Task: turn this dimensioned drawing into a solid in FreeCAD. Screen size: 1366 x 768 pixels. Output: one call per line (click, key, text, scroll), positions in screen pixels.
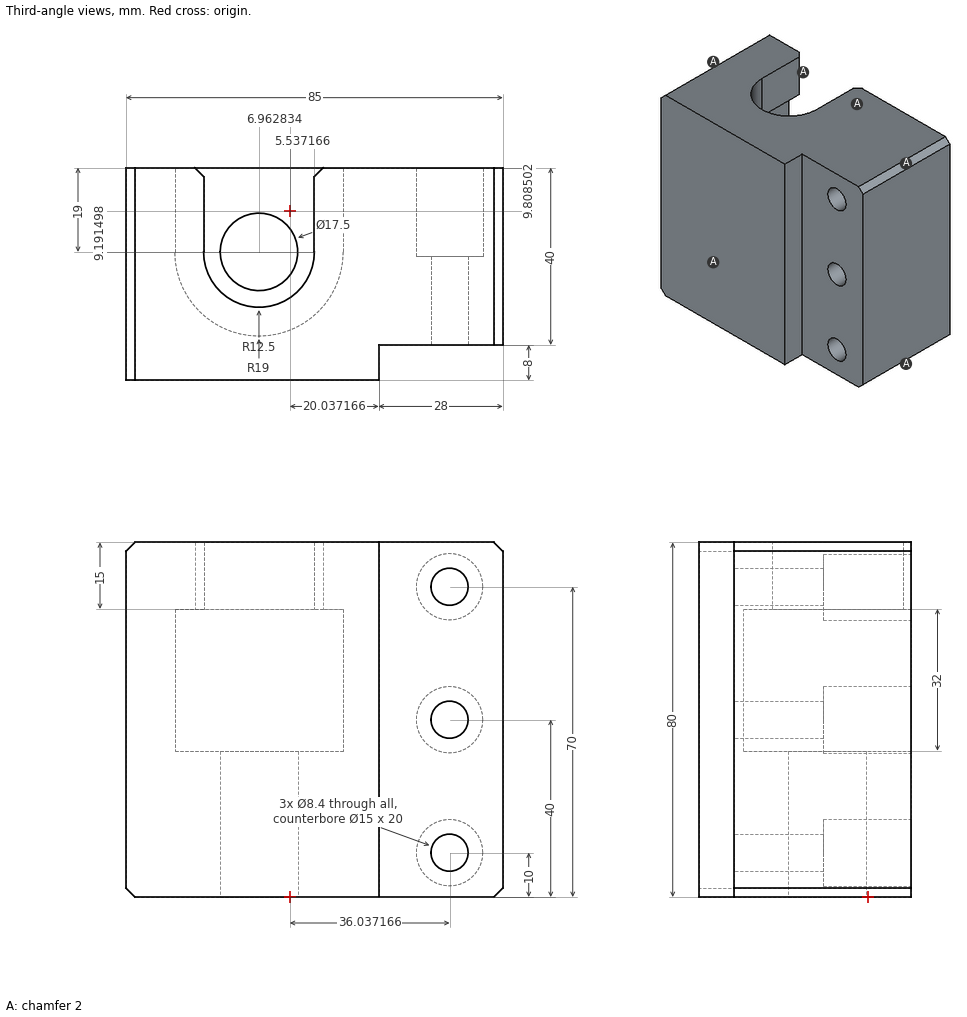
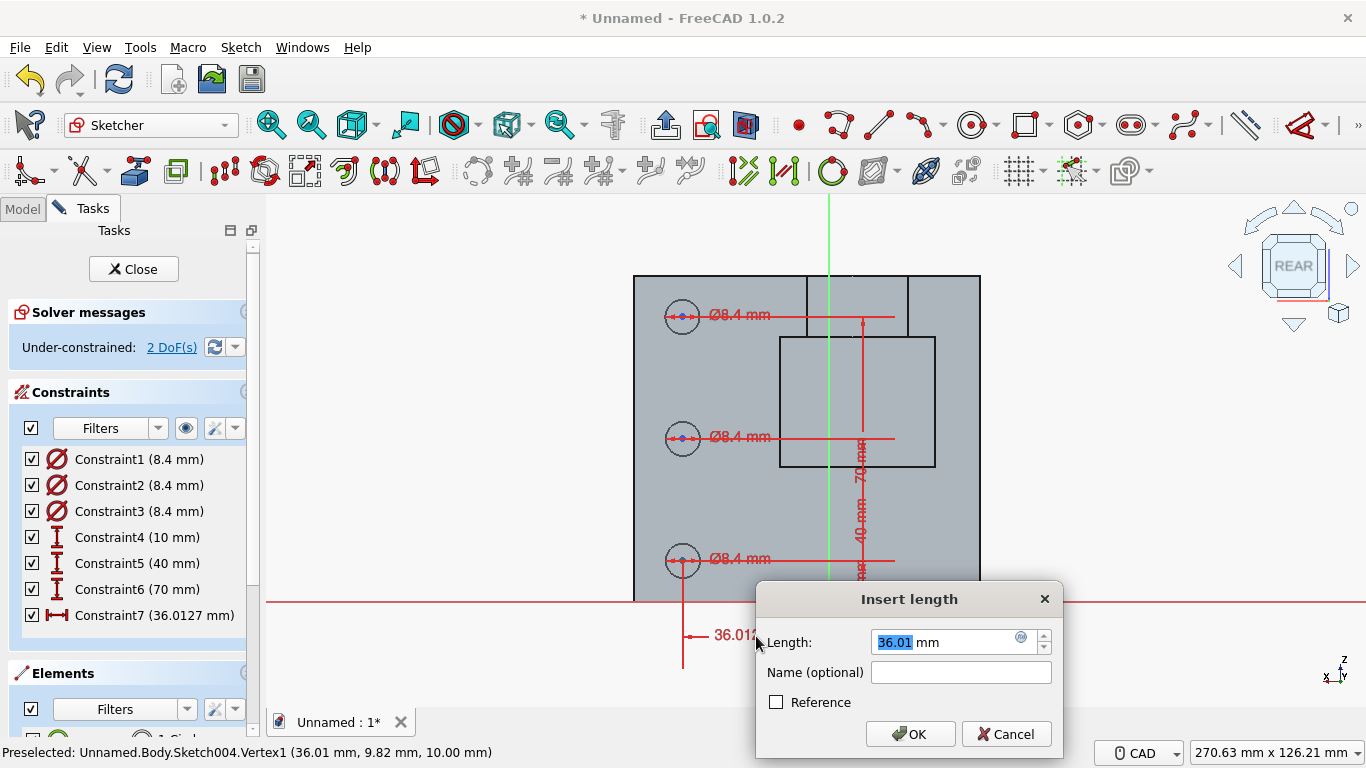
text(36.037166)
key(Return)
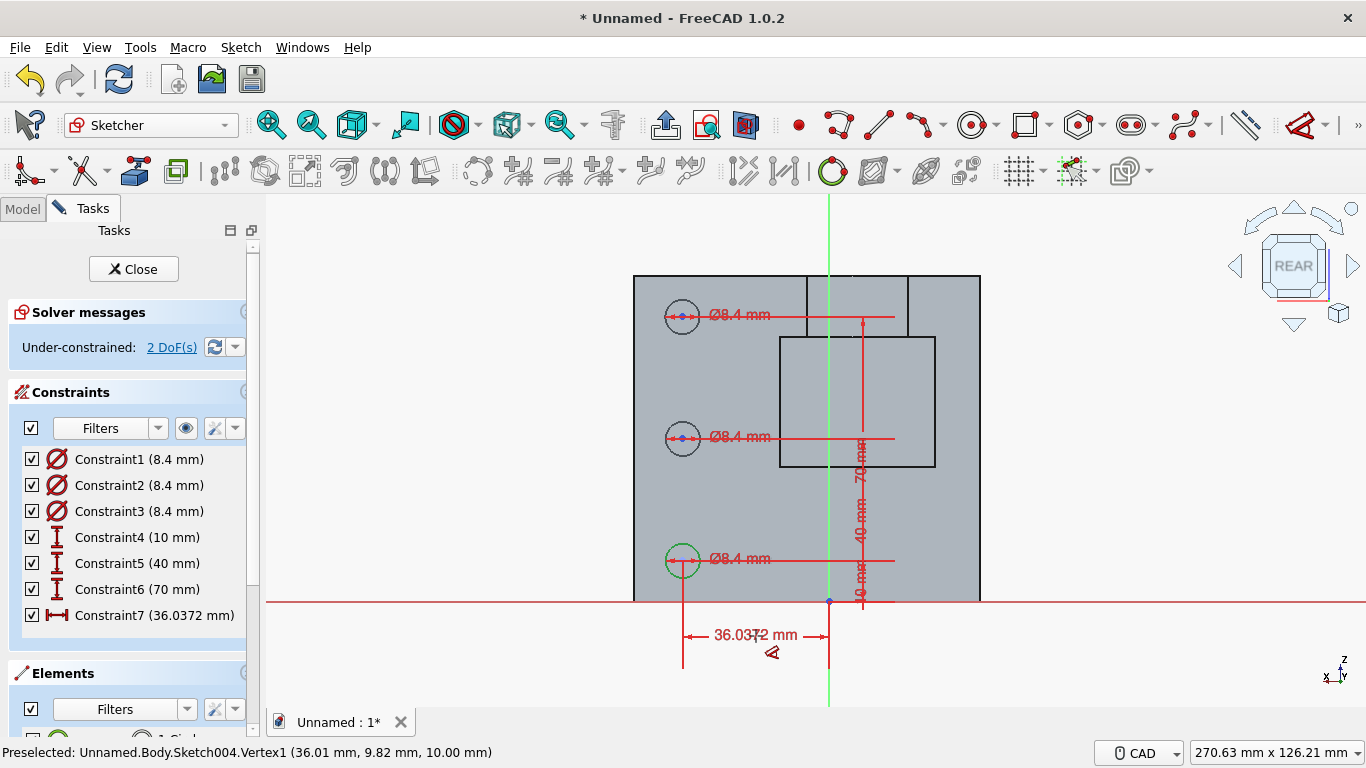
click(683, 439)
click(756, 405)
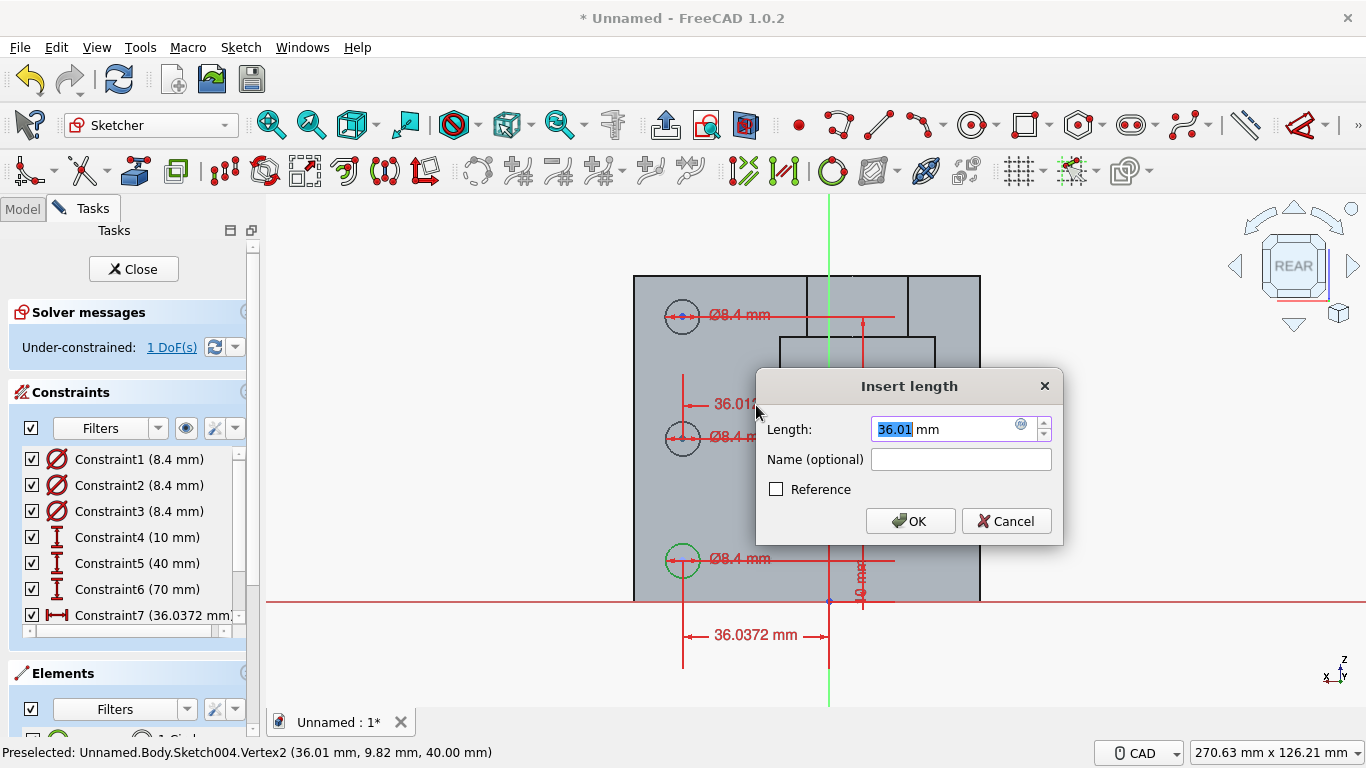
text(36.037166)
key(Return)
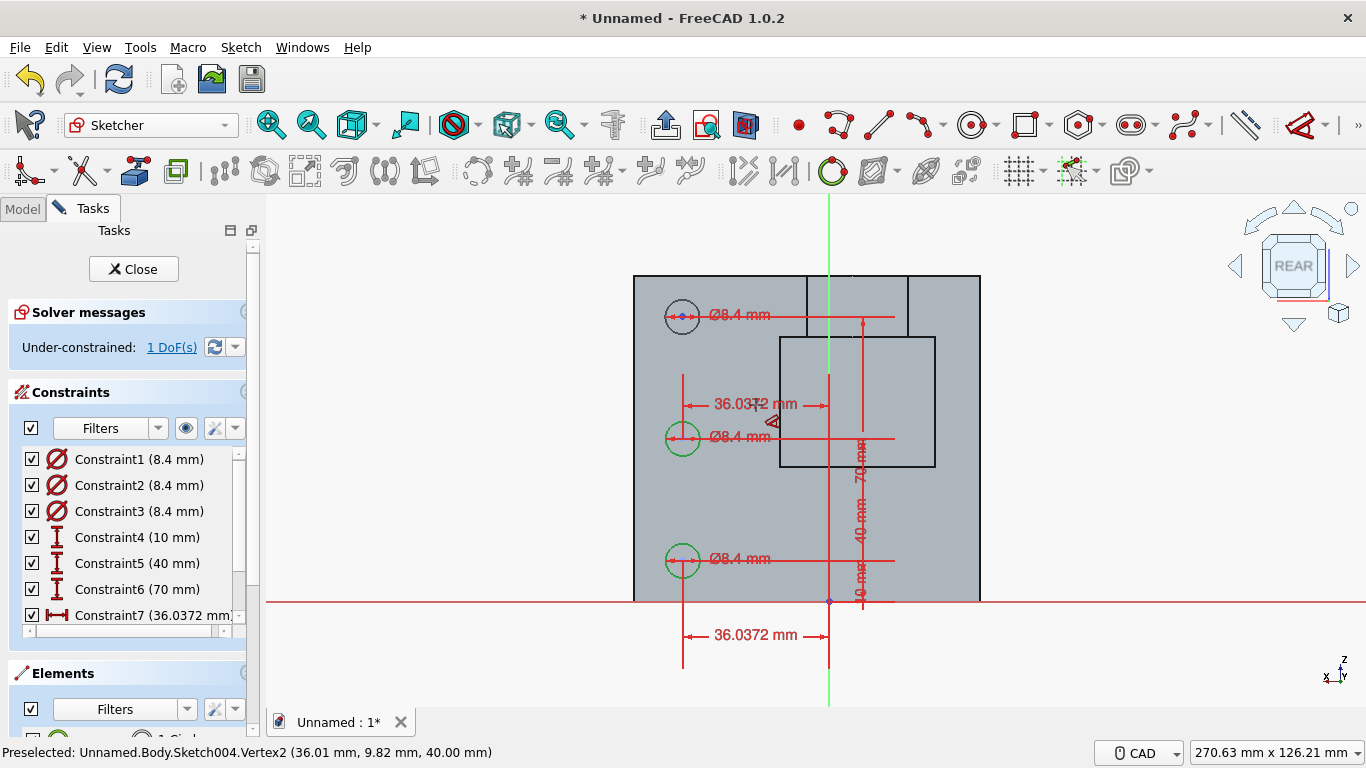
click(682, 317)
click(756, 283)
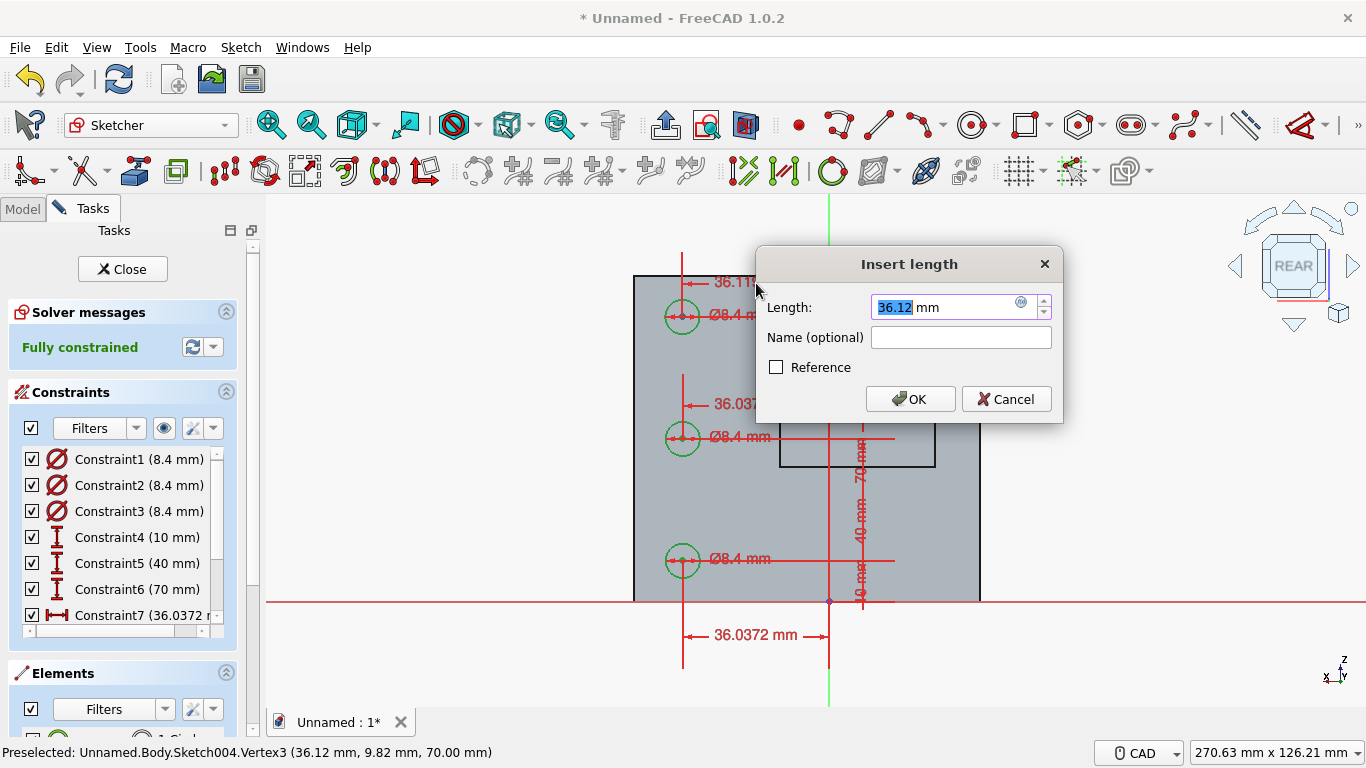
text(36.037166)
key(Return)
key(Escape)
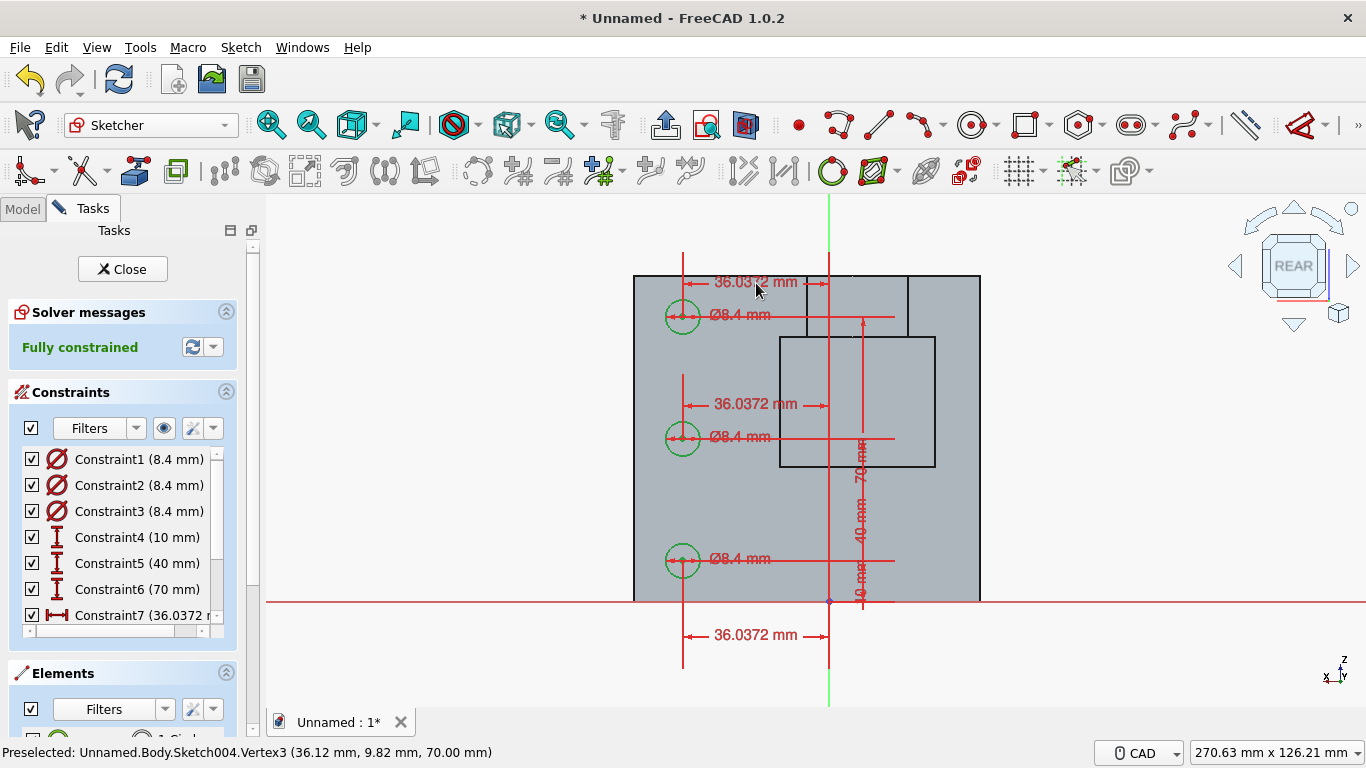
click(123, 269)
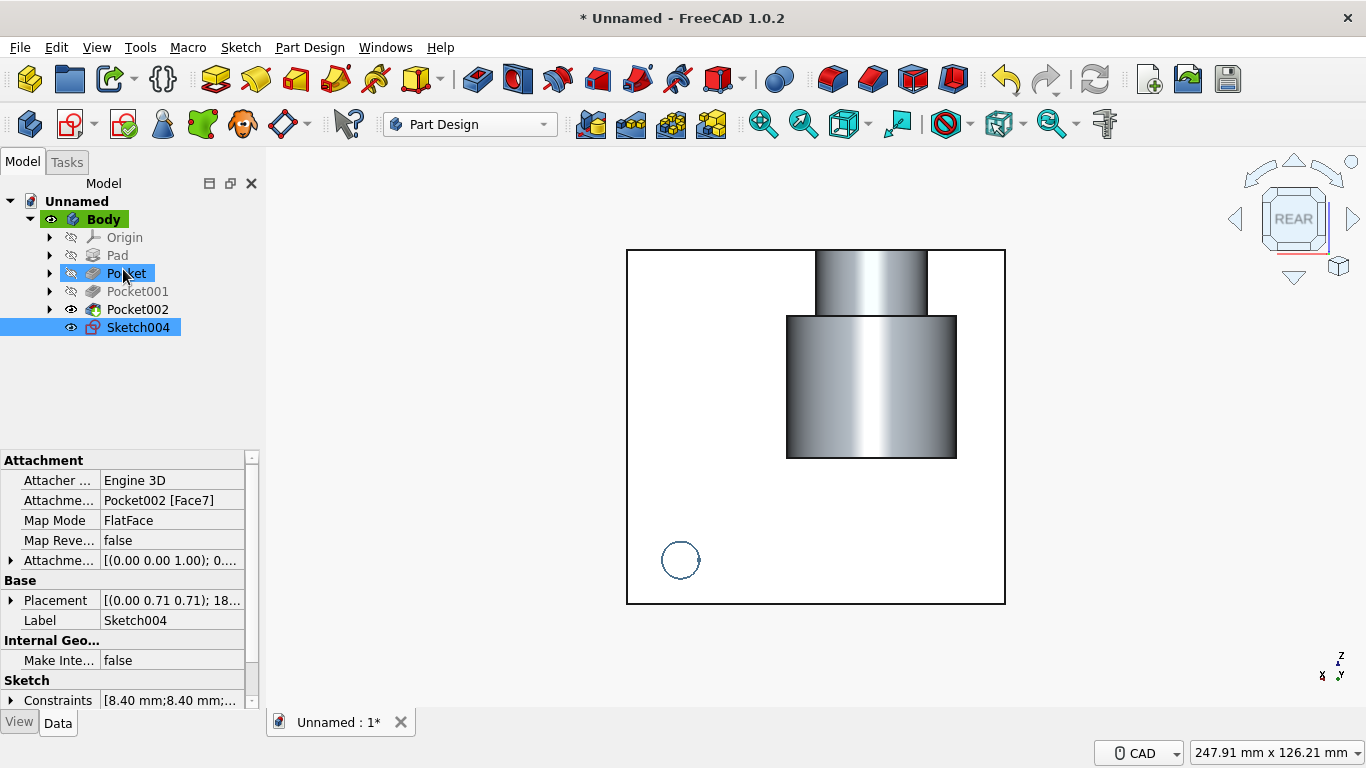
click(518, 80)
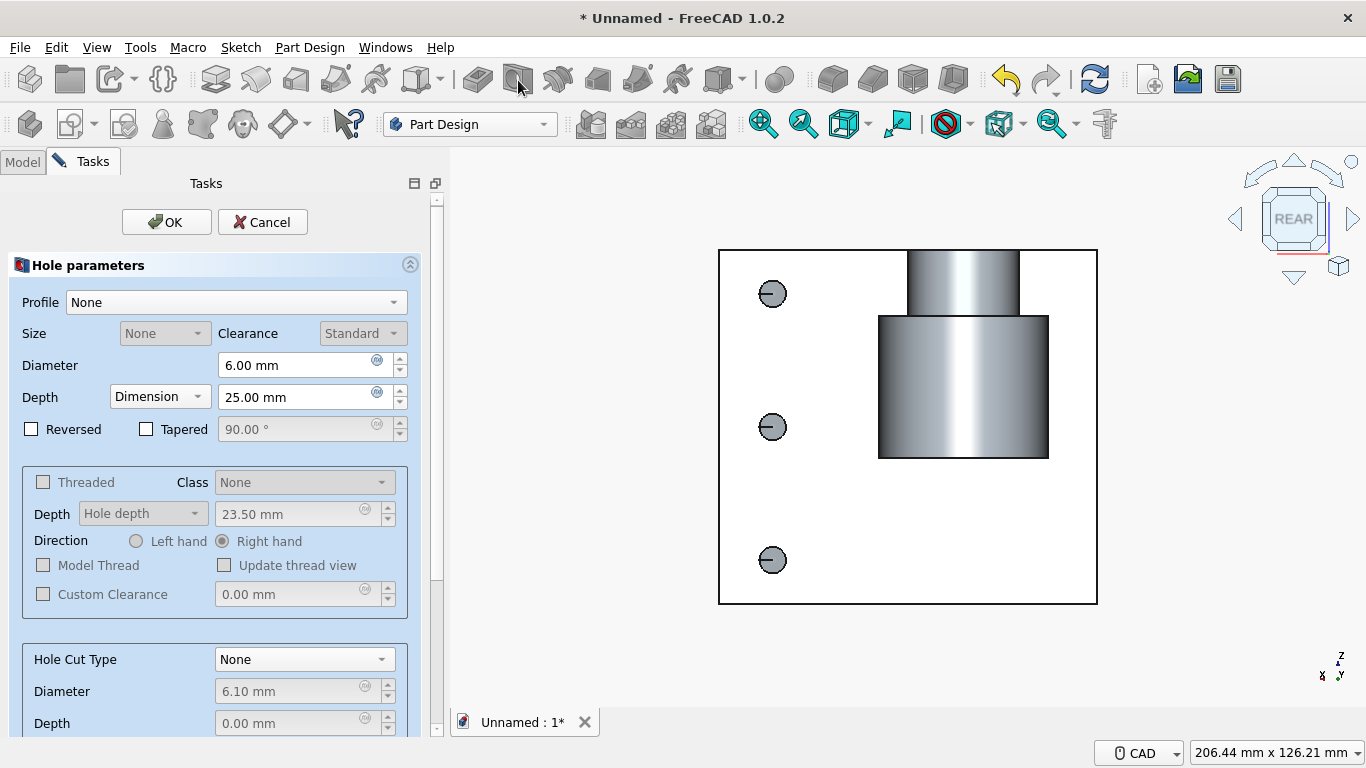
triple_click(305, 365)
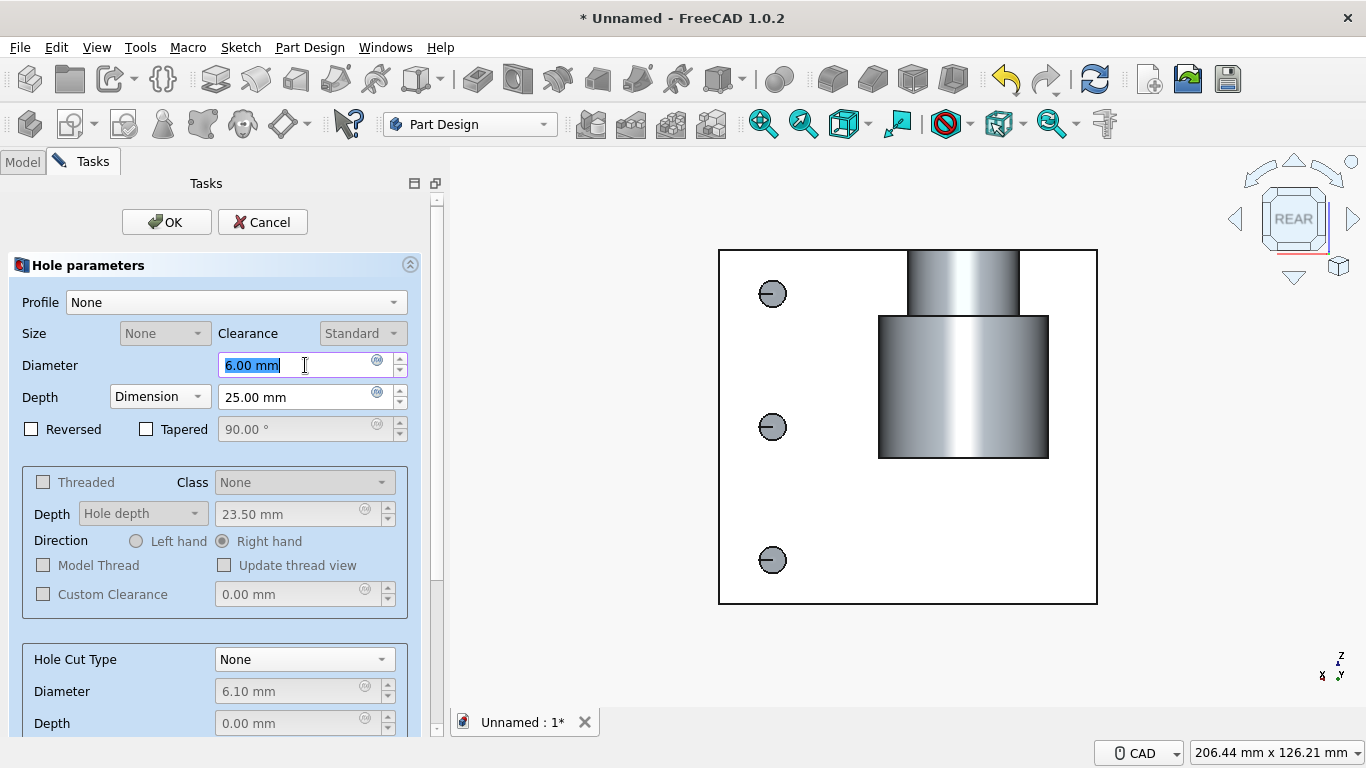
text(8.4)
key(Tab)